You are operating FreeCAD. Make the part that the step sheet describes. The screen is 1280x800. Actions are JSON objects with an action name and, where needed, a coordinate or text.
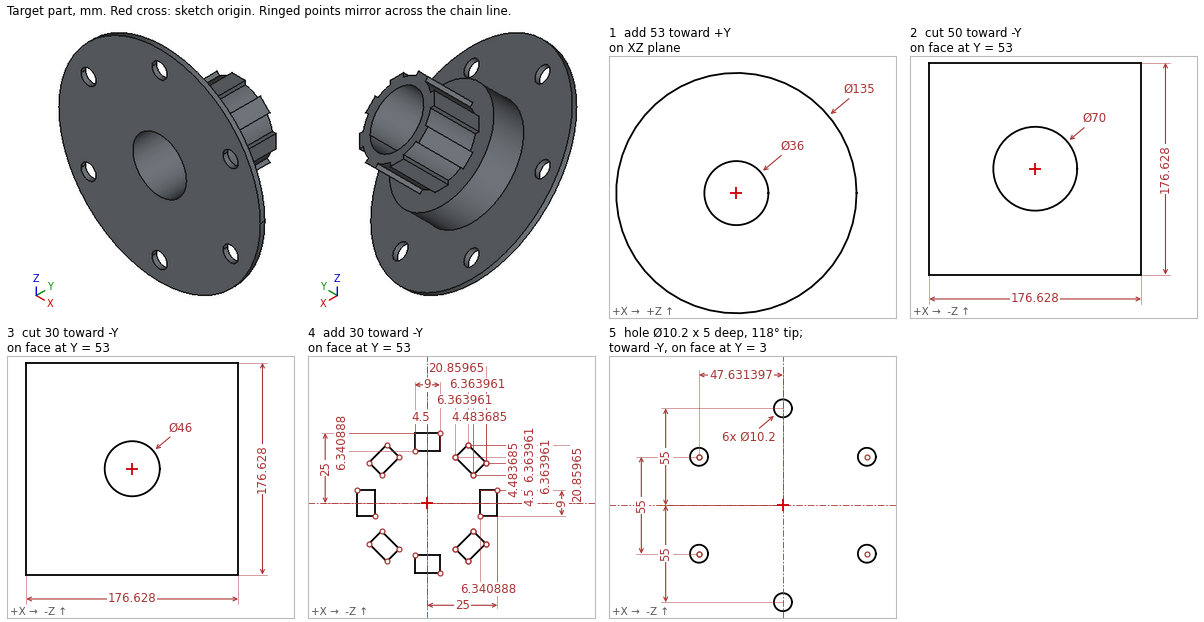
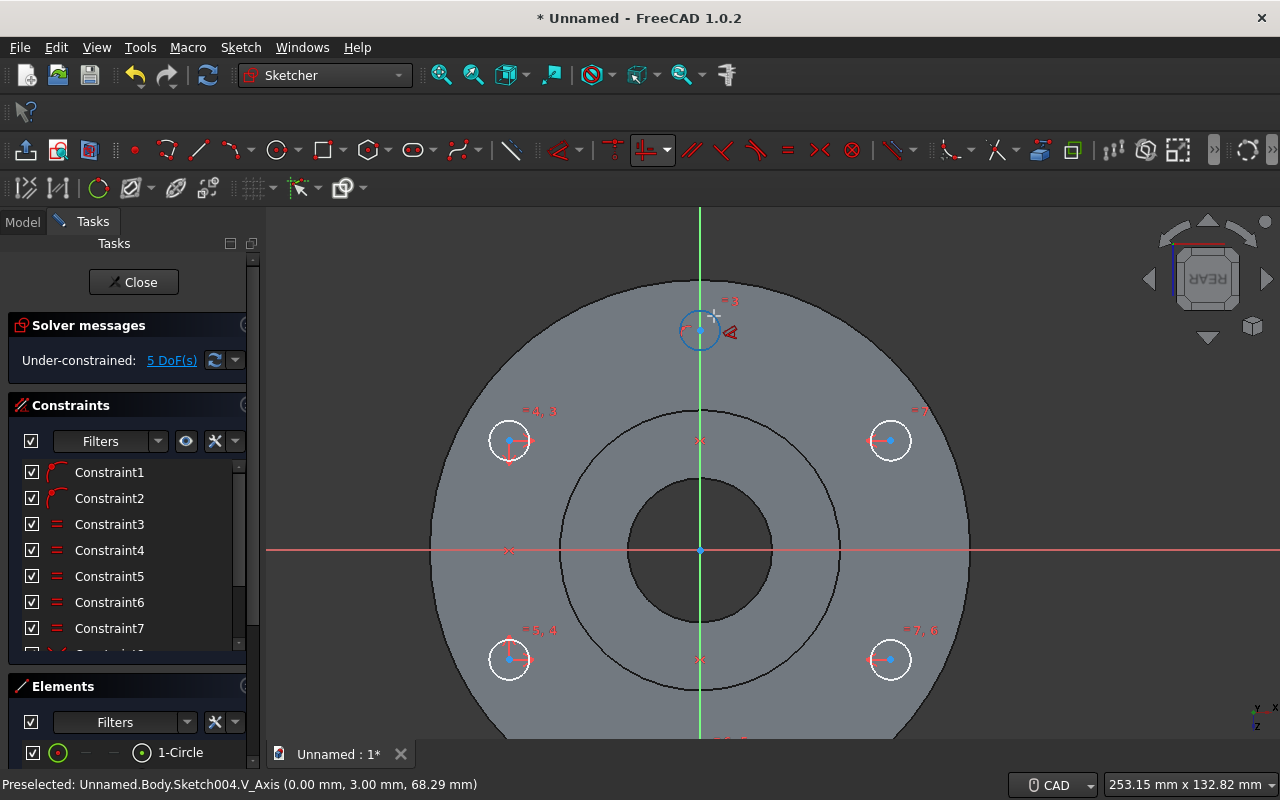
{"action": "left_click", "coordinate": [714, 316]}
{"action": "left_click", "coordinate": [736, 293]}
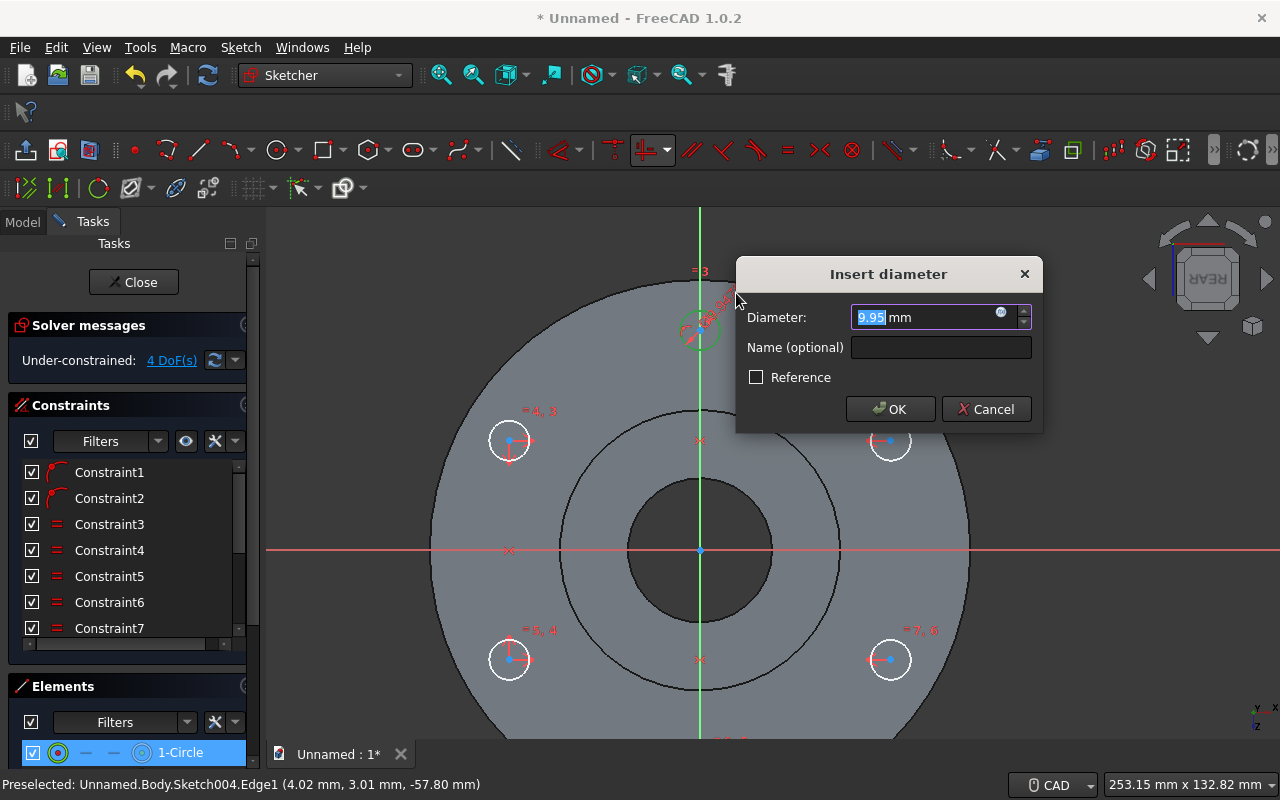
{"action": "type", "text": "10.2"}
{"action": "key", "text": "Return"}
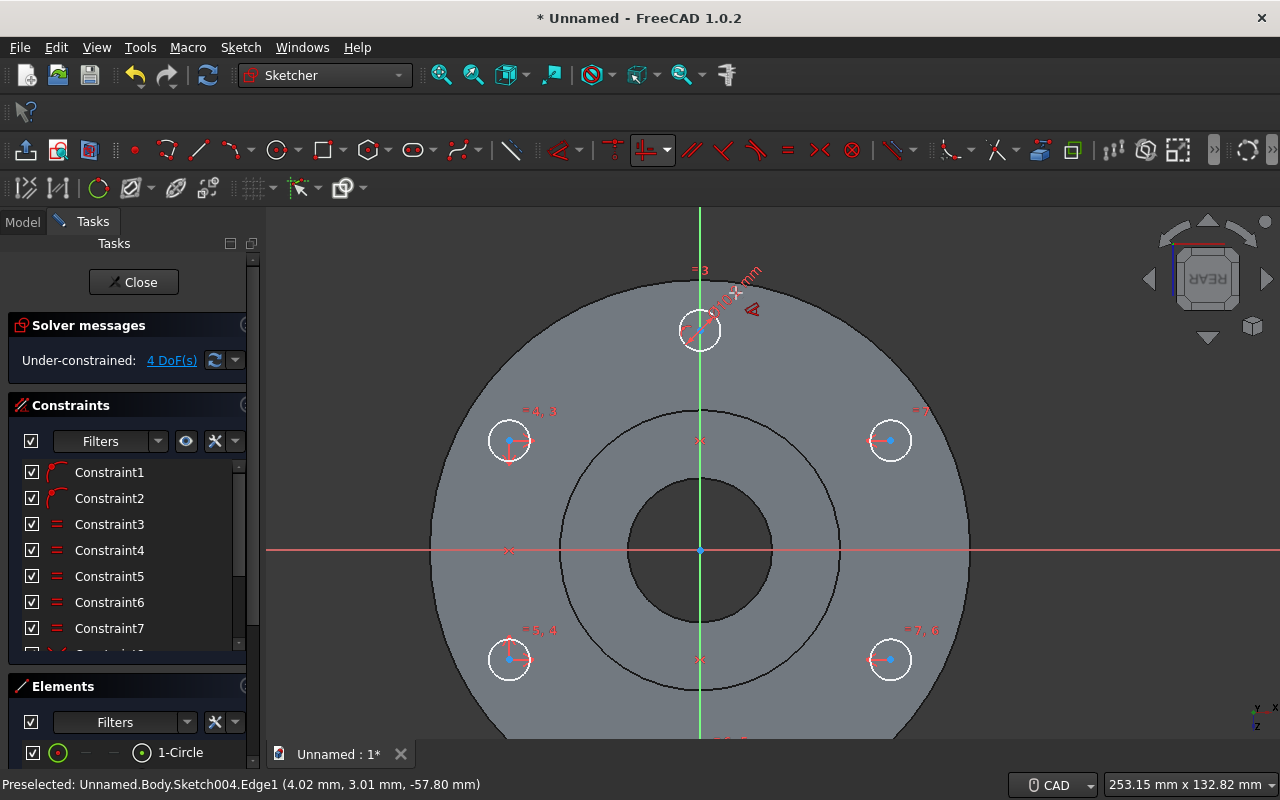
{"action": "left_click", "coordinate": [700, 330]}
{"action": "left_click", "coordinate": [734, 440]}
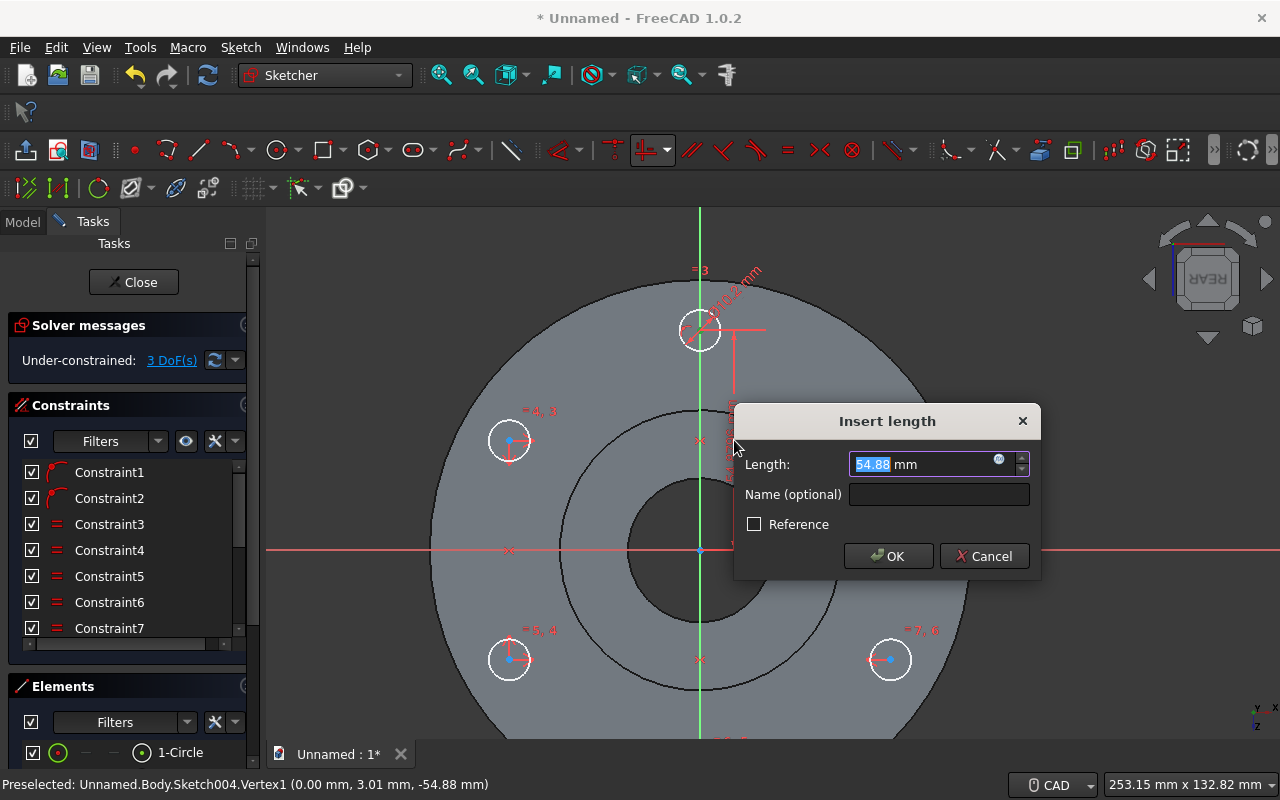
{"action": "type", "text": "55"}
{"action": "key", "text": "Return"}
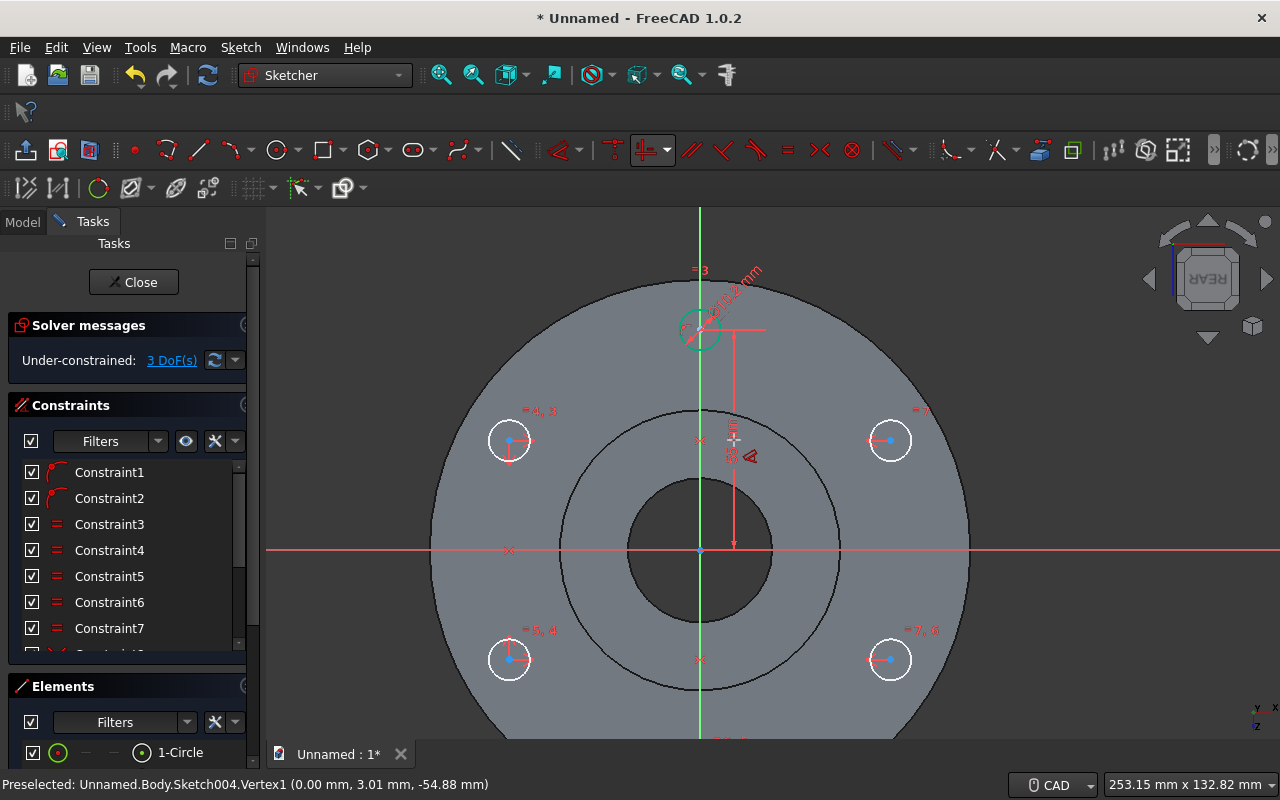
{"action": "scroll", "coordinate": [714, 316], "scroll_direction": "down", "scroll_amount": 2}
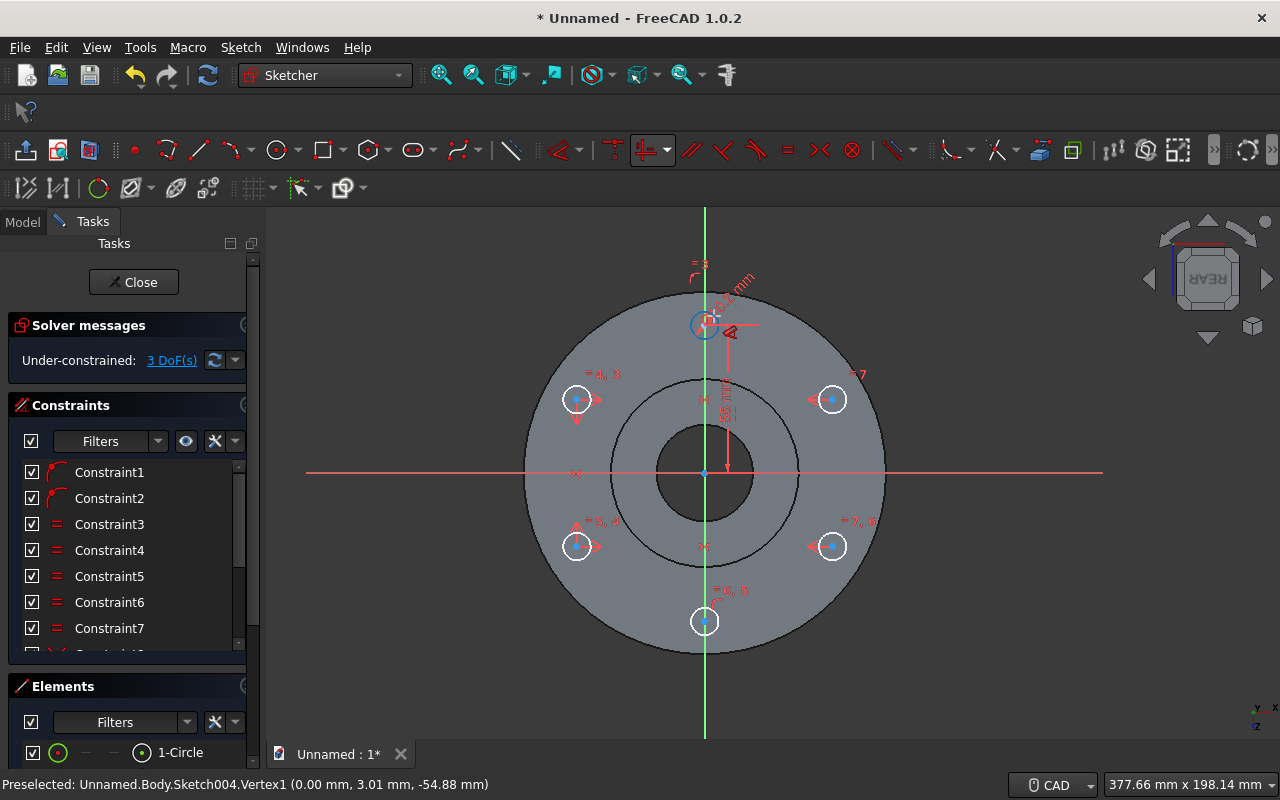
{"action": "left_click", "coordinate": [705, 622]}
{"action": "left_click", "coordinate": [739, 547]}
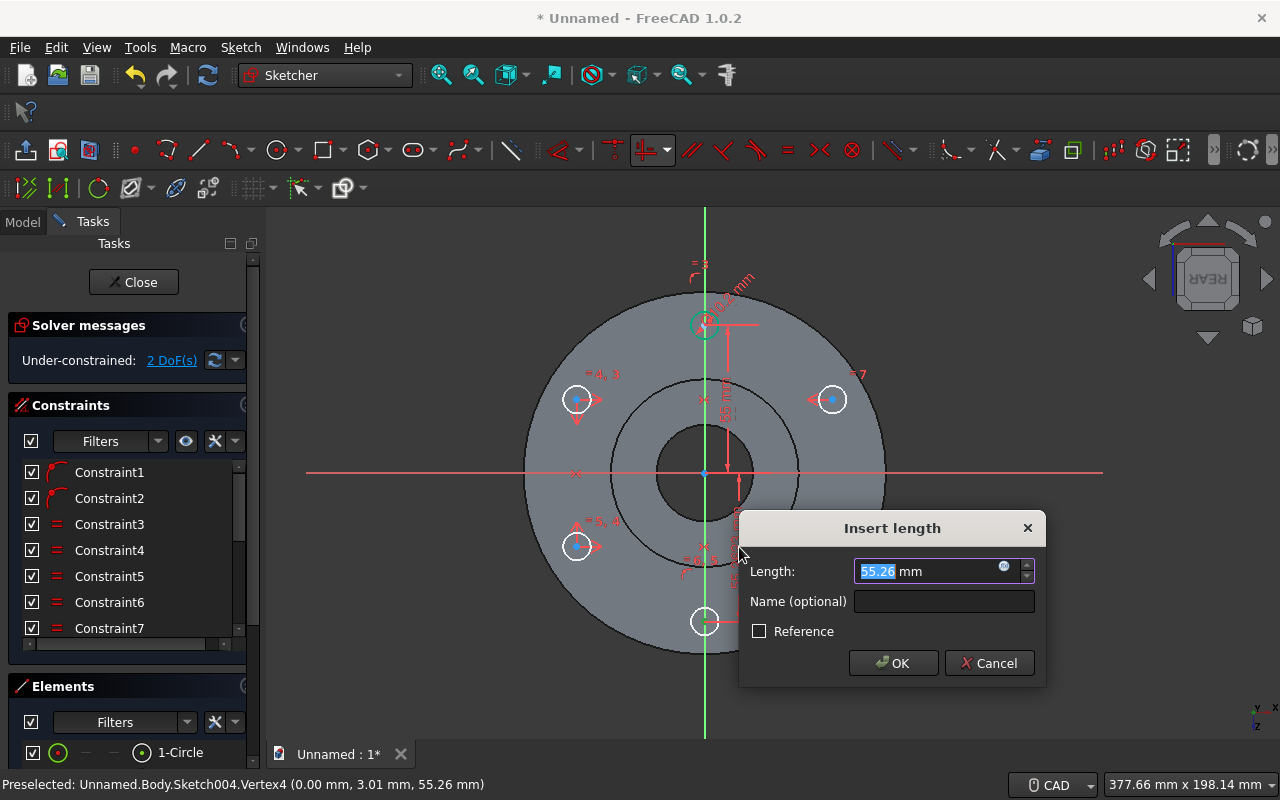
{"action": "type", "text": "55"}
{"action": "key", "text": "Return"}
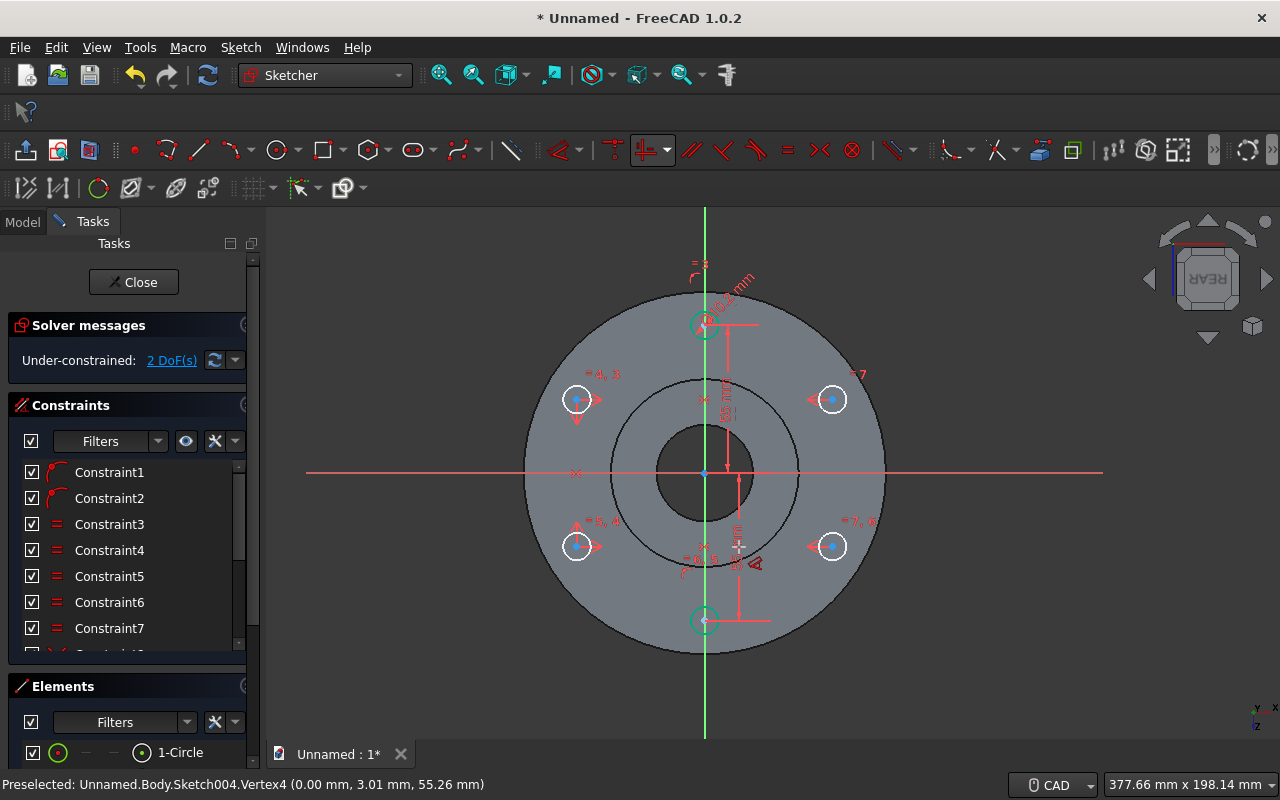
{"action": "left_click", "coordinate": [577, 400]}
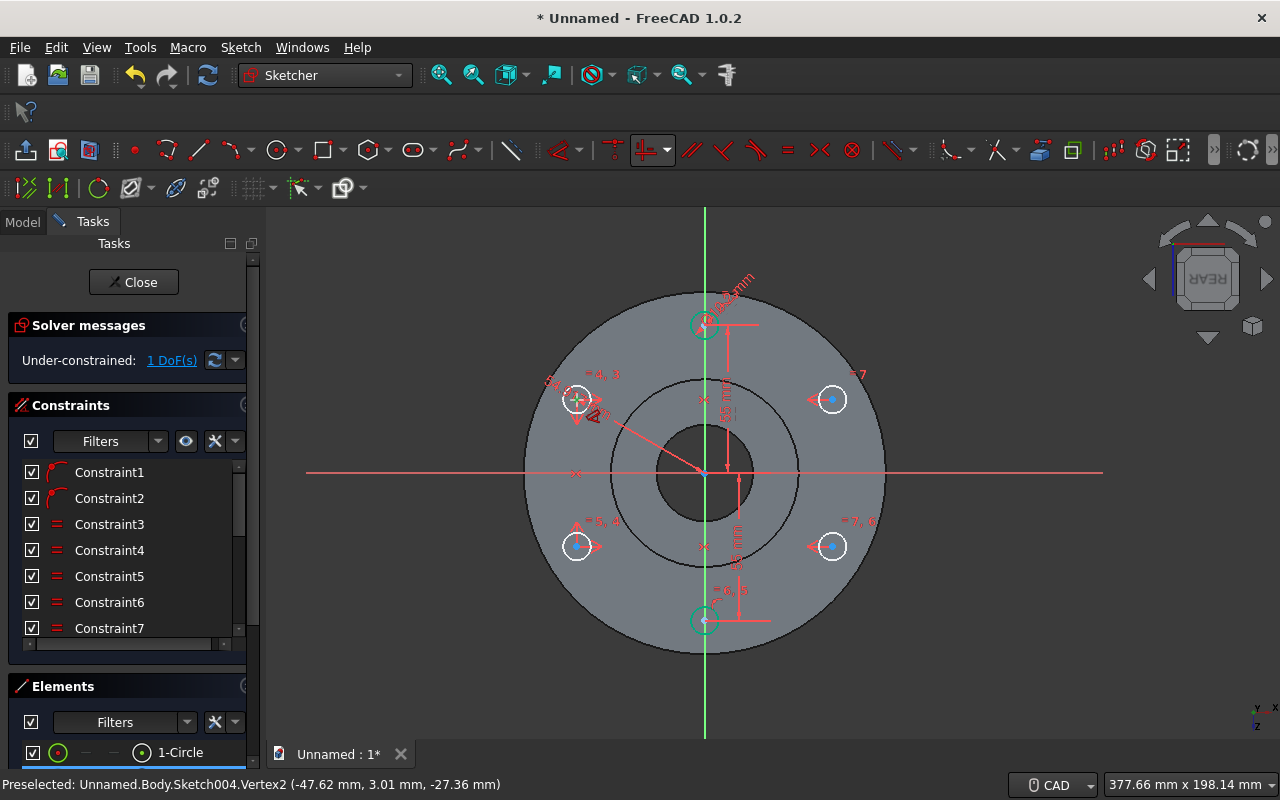
{"action": "left_click", "coordinate": [577, 547]}
{"action": "left_click", "coordinate": [543, 439]}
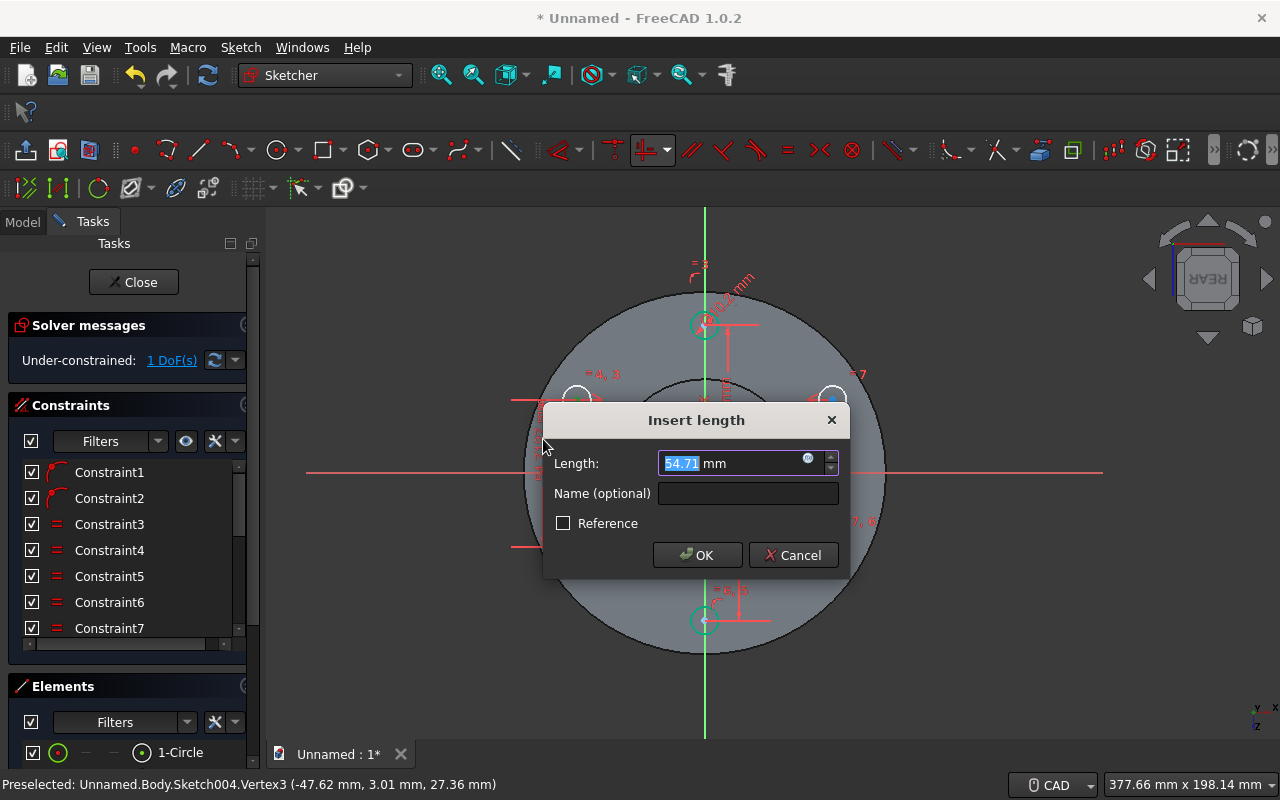
{"action": "type", "text": "55"}
{"action": "key", "text": "Return"}